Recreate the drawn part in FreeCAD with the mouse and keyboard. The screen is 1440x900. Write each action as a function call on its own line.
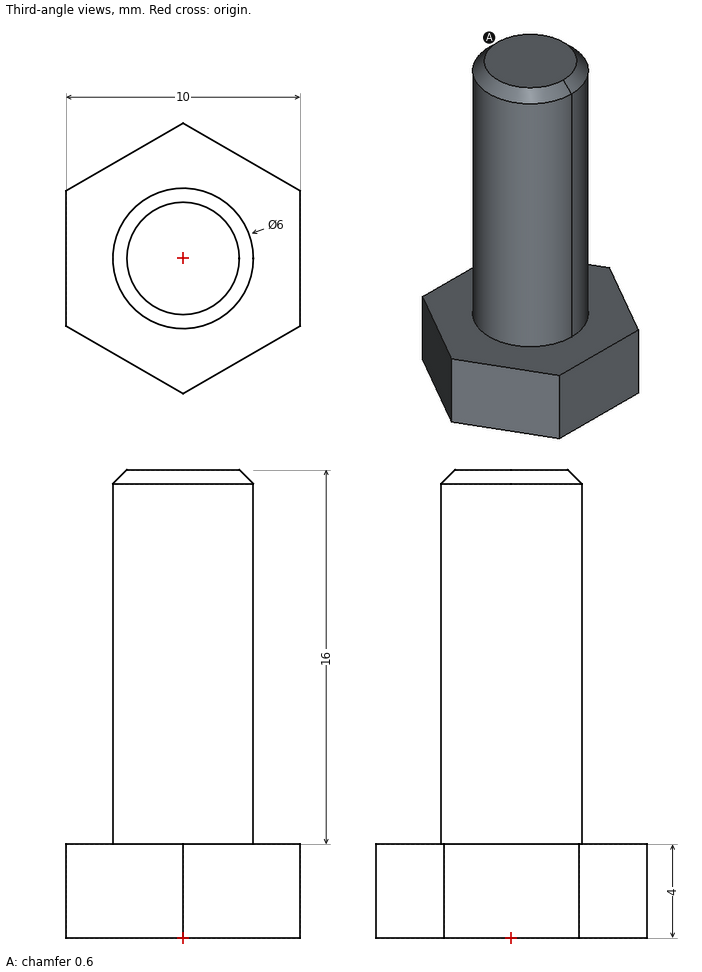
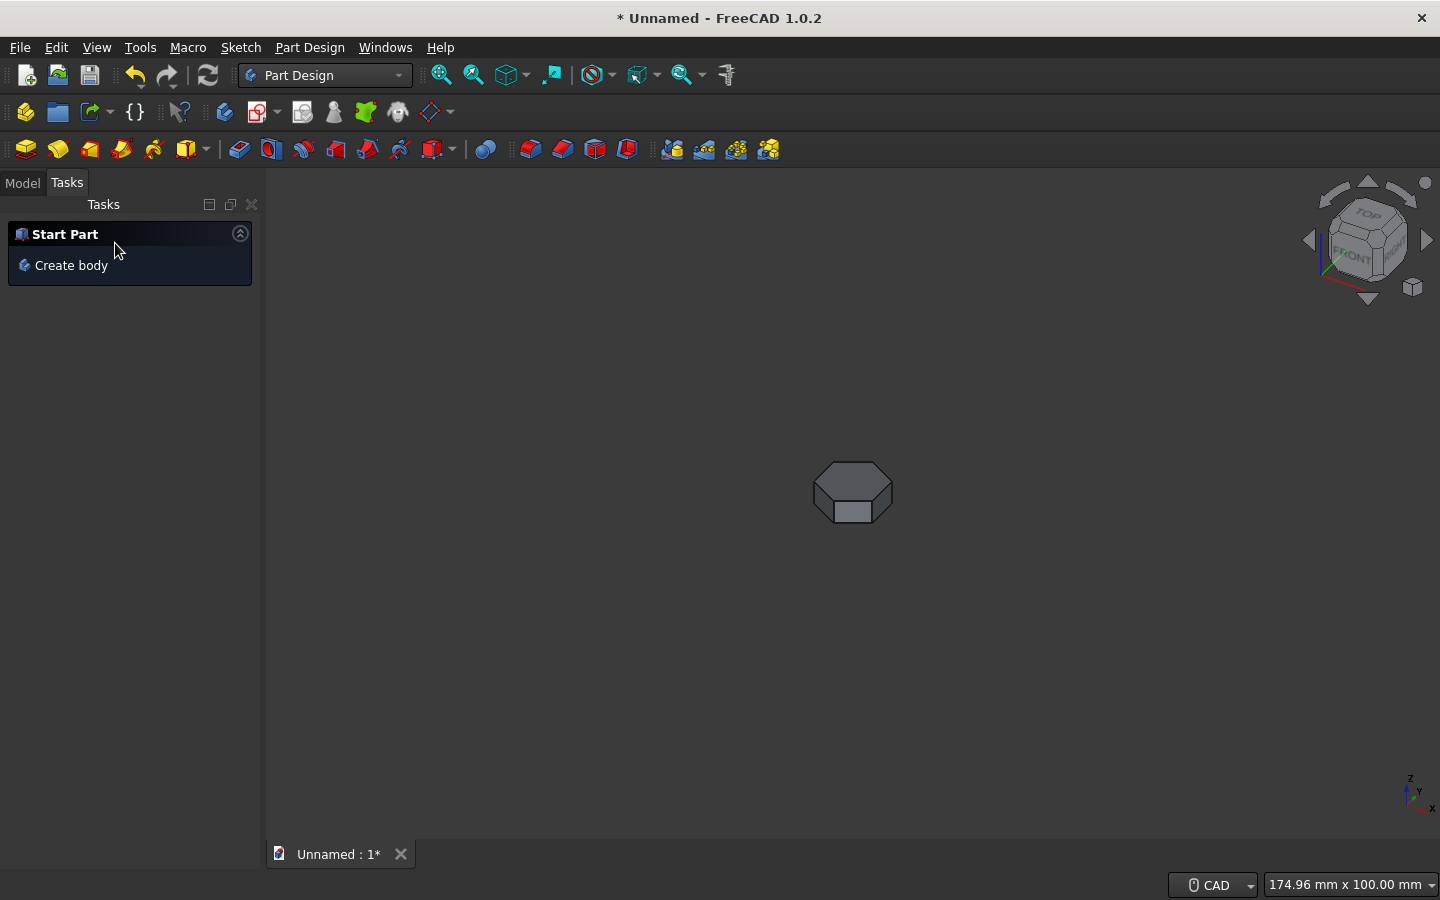
click(442, 76)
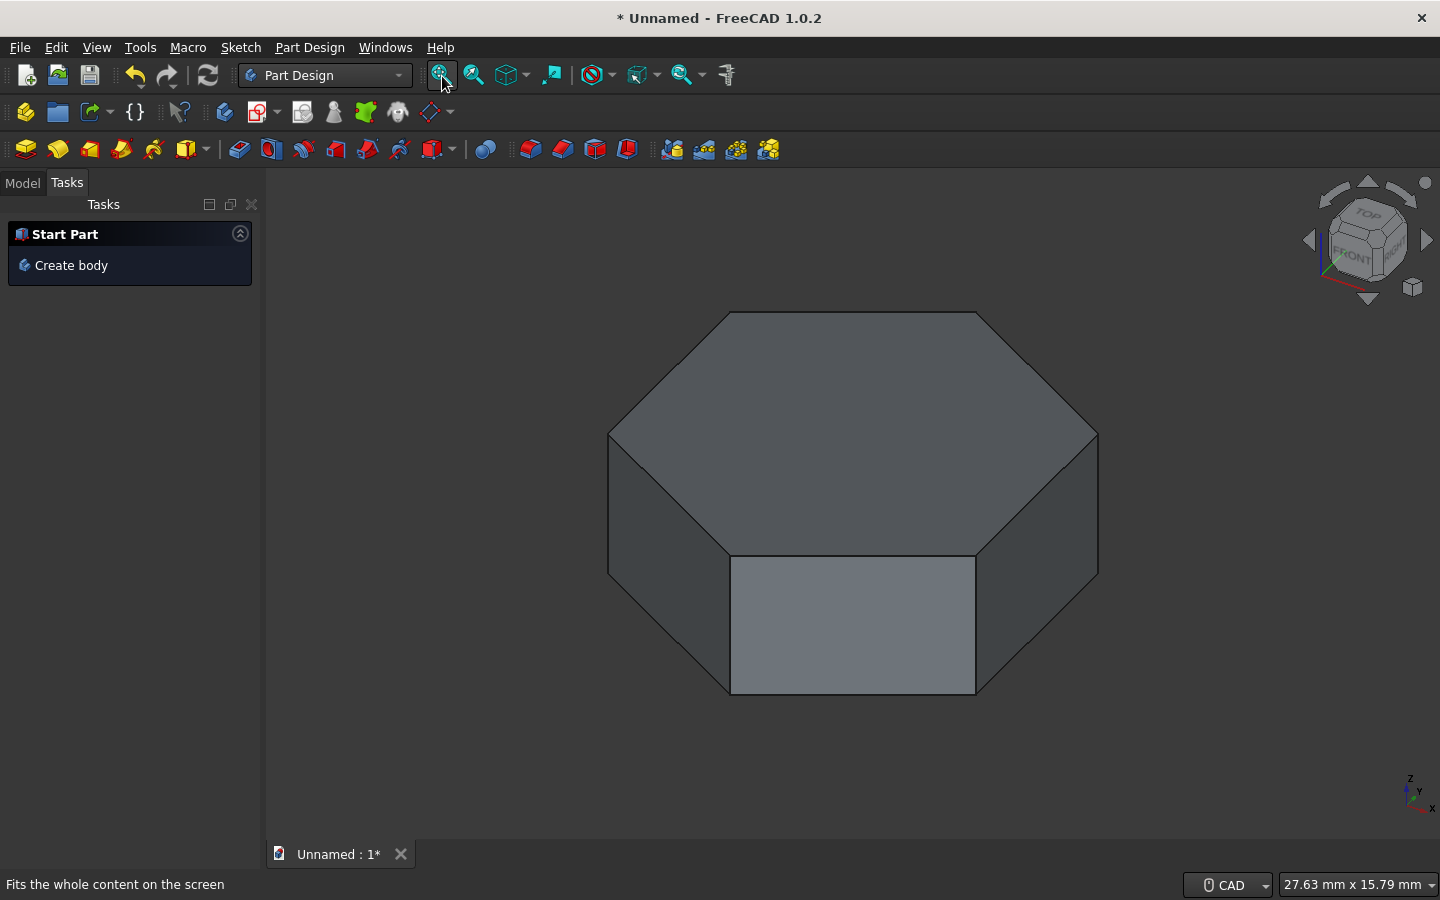
click(853, 433)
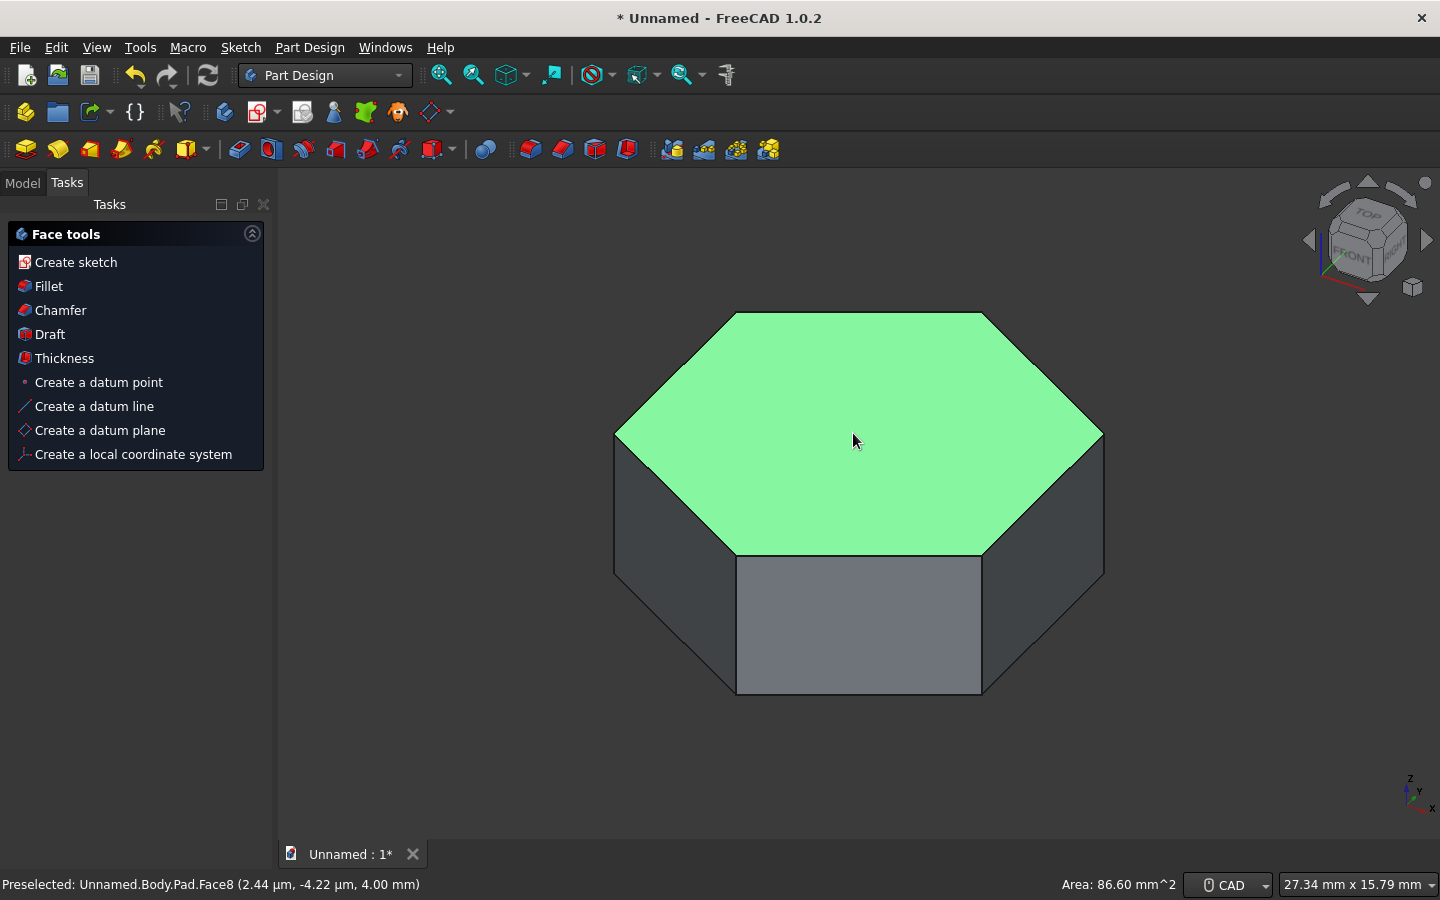
click(258, 112)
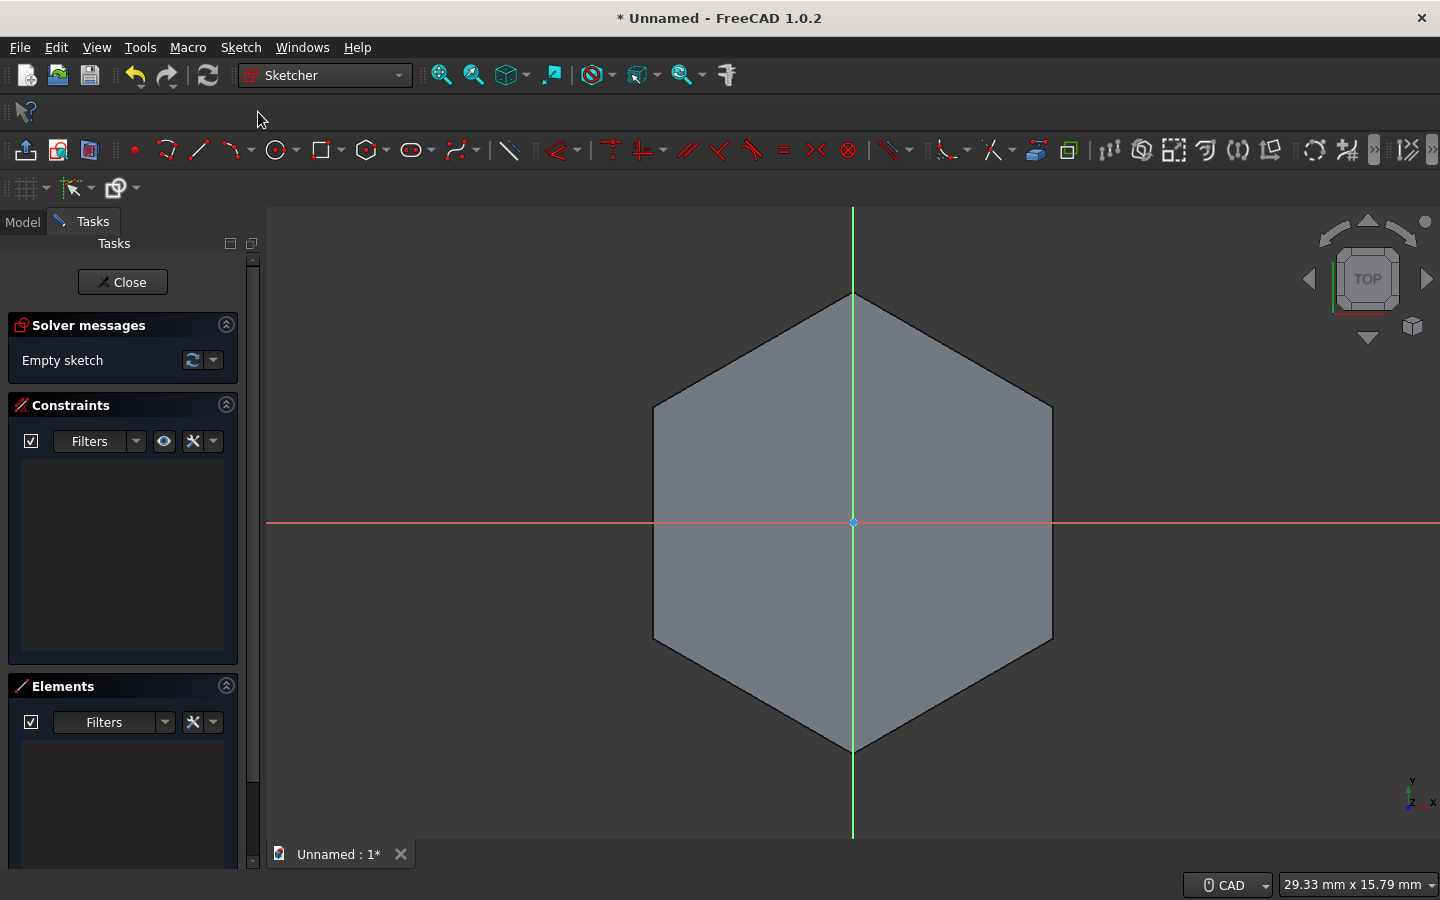
scroll(936, 523, up, 3)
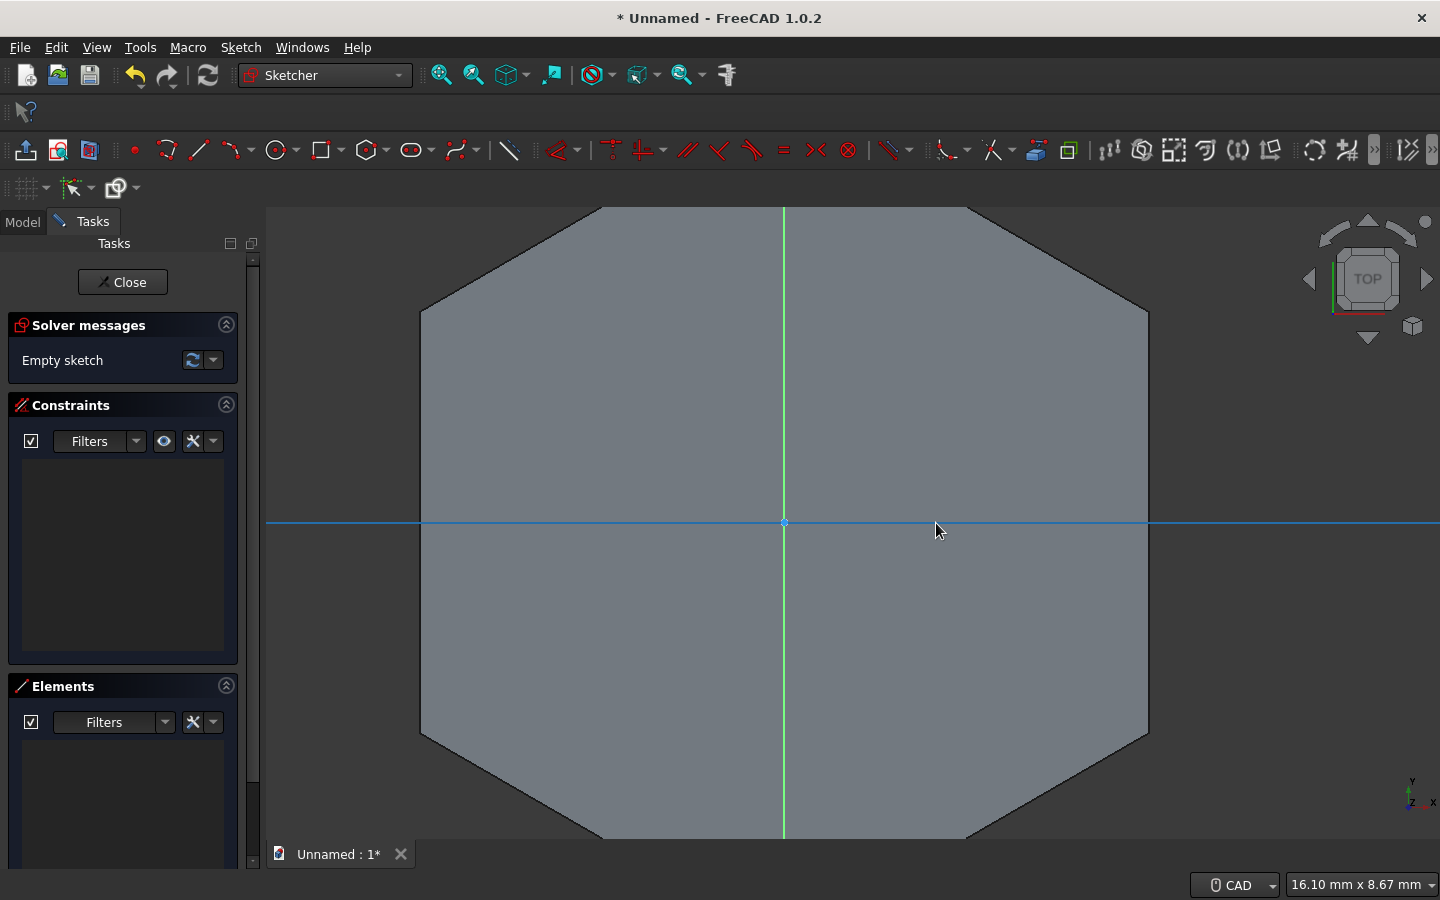
key(g)
key(c)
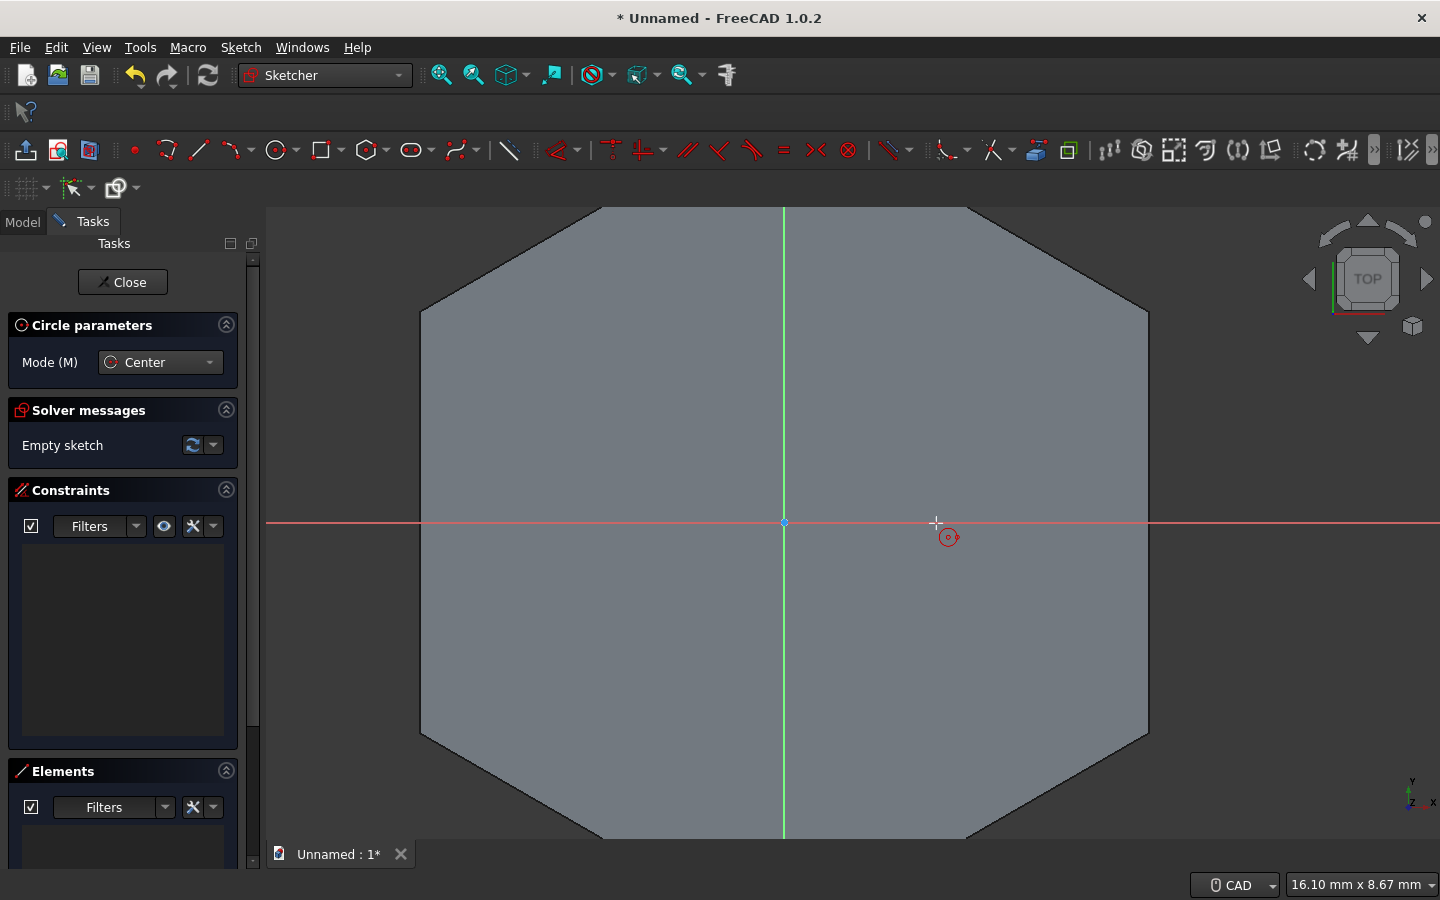
click(784, 523)
move(939, 368)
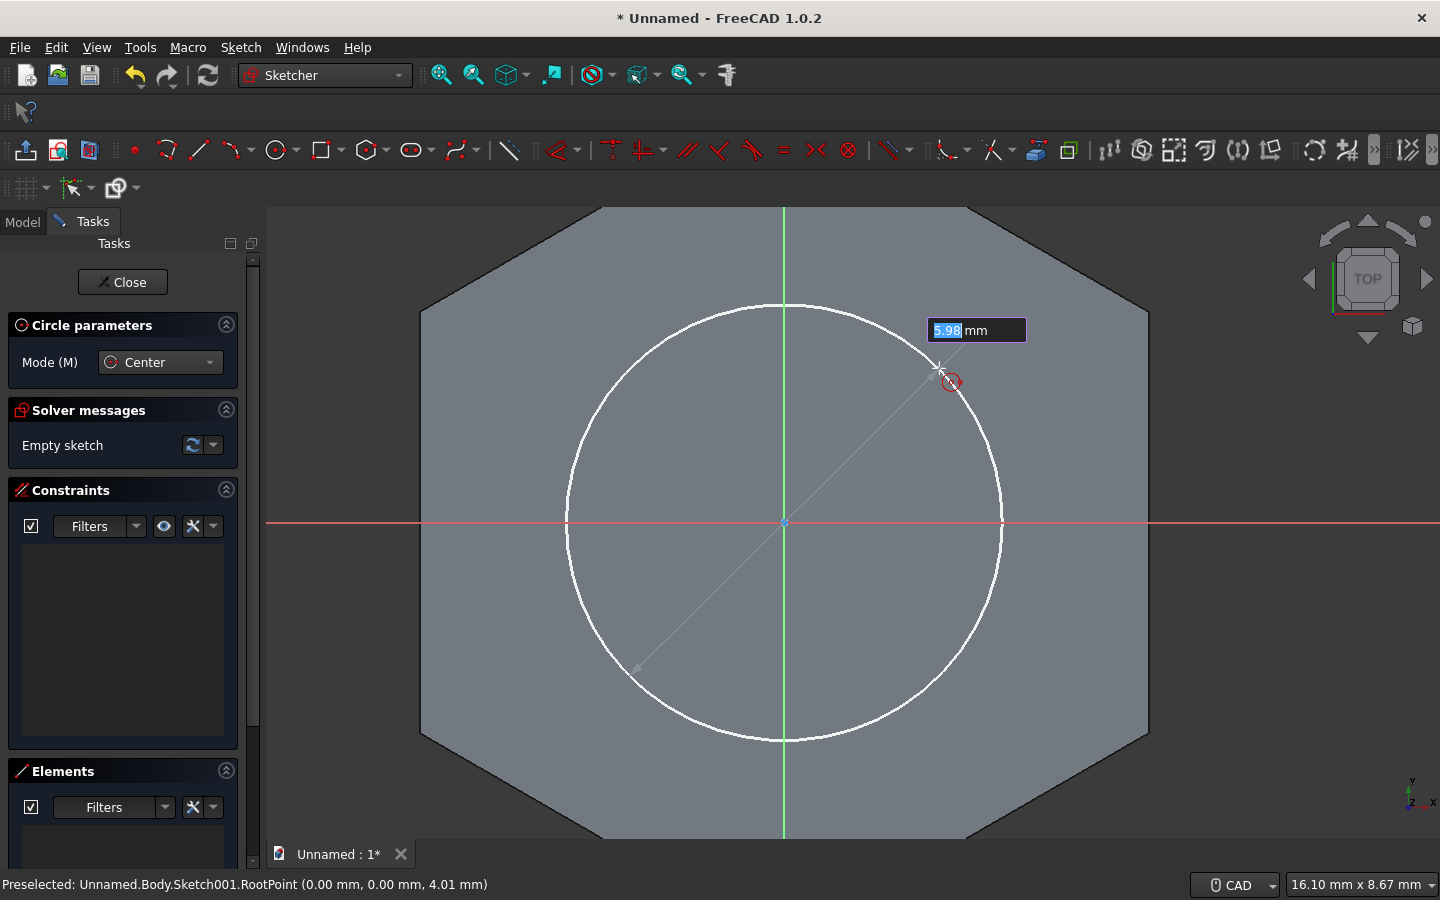
text(6)
key(Return)
key(Escape)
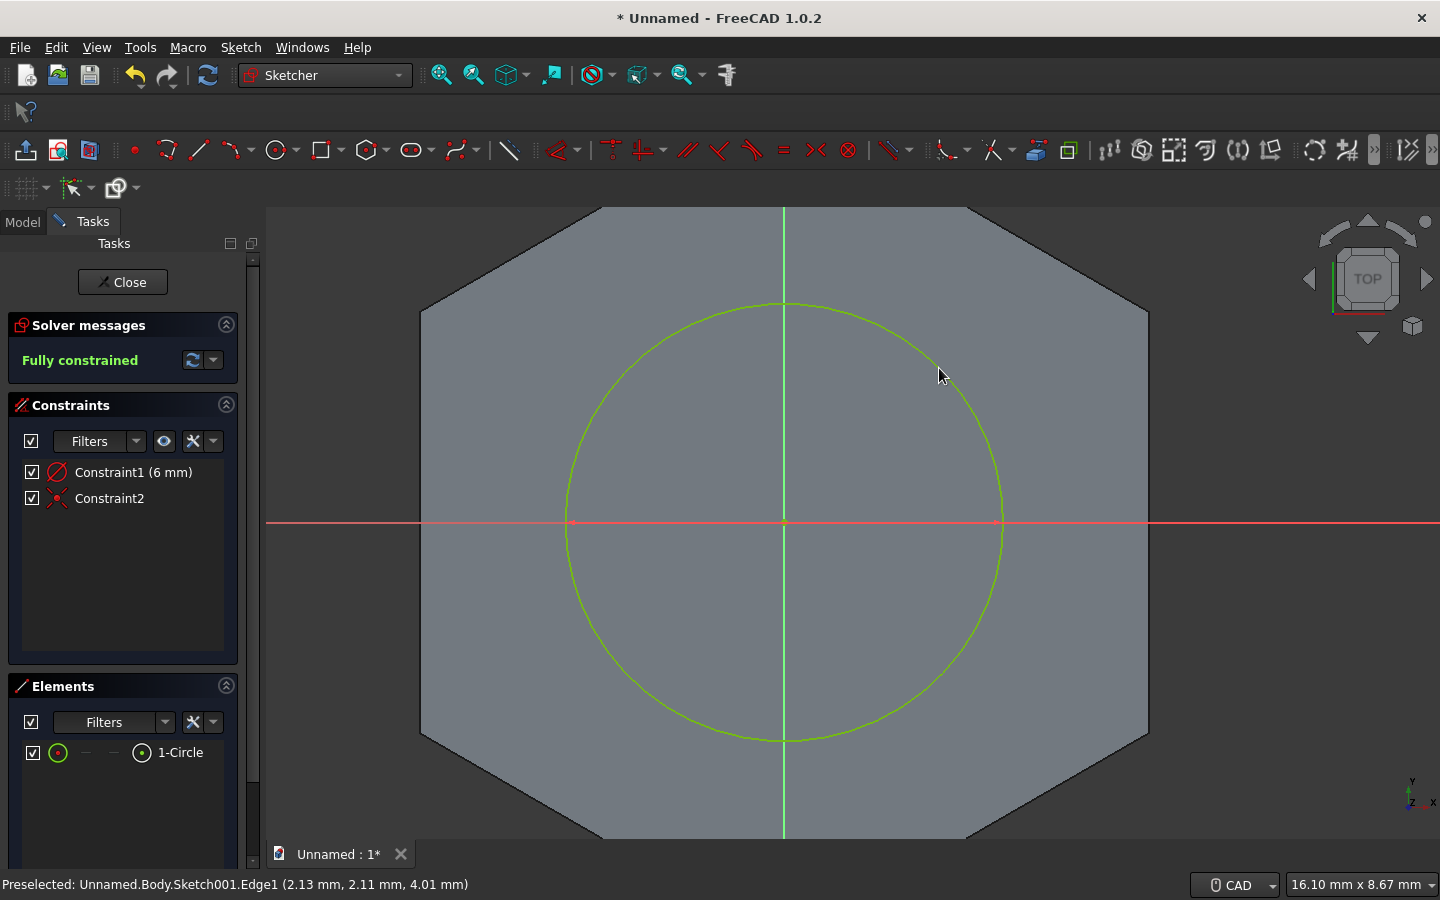
click(123, 282)